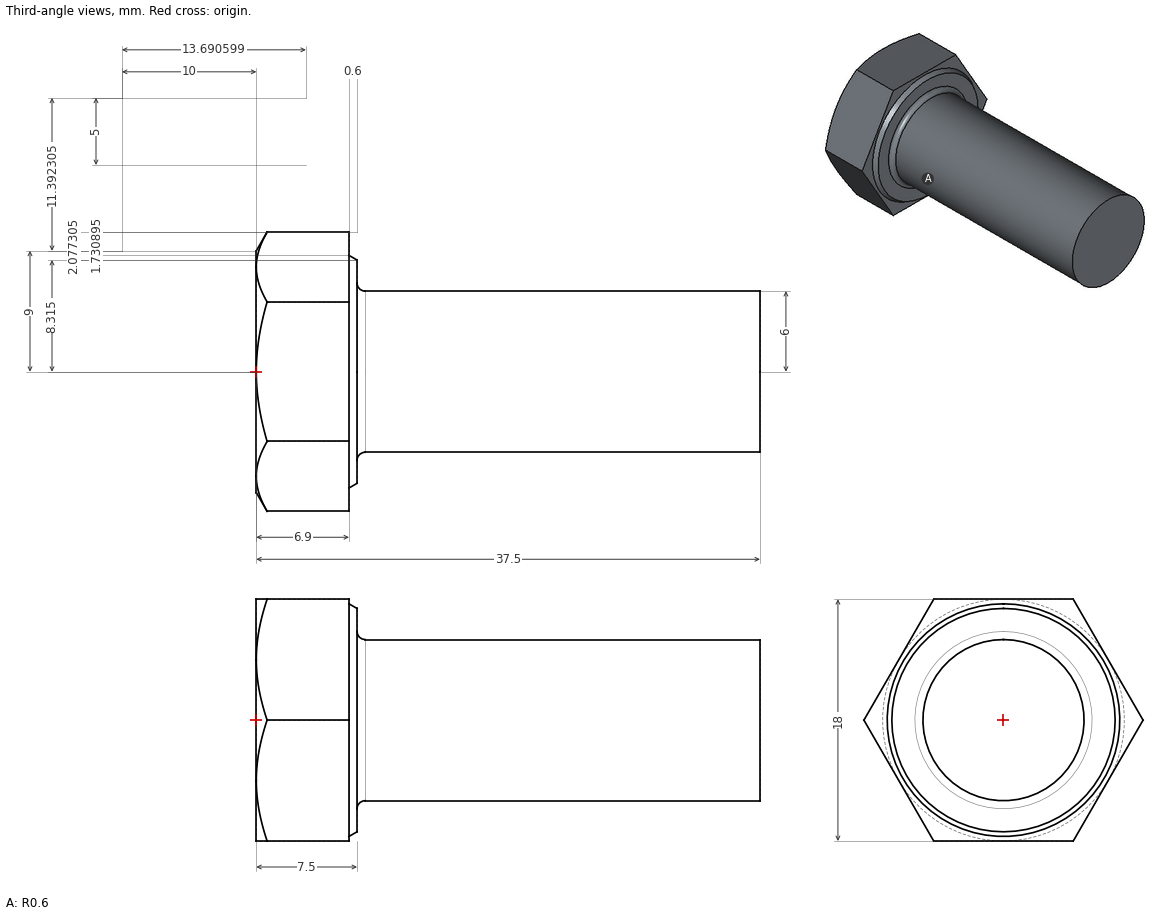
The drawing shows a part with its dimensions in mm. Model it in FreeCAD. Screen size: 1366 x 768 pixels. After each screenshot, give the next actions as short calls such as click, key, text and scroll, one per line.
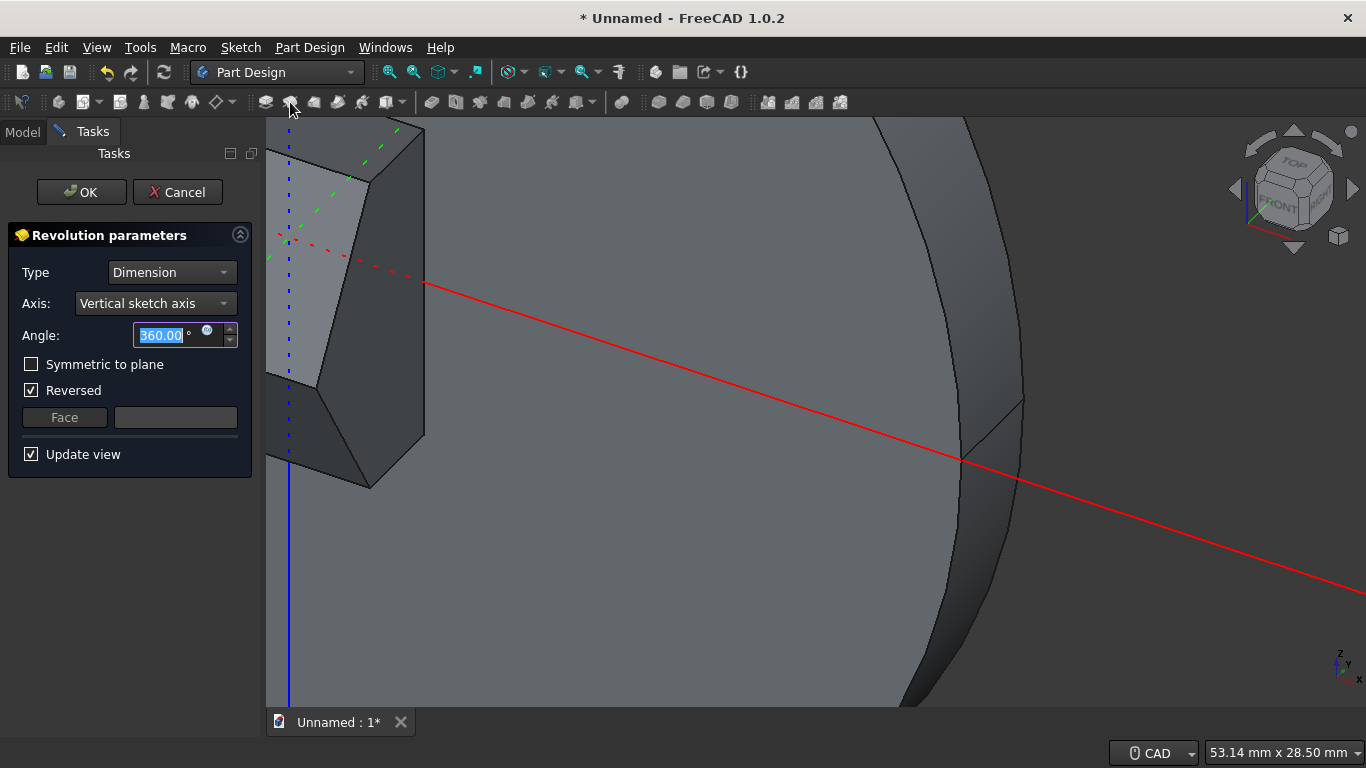
click(156, 304)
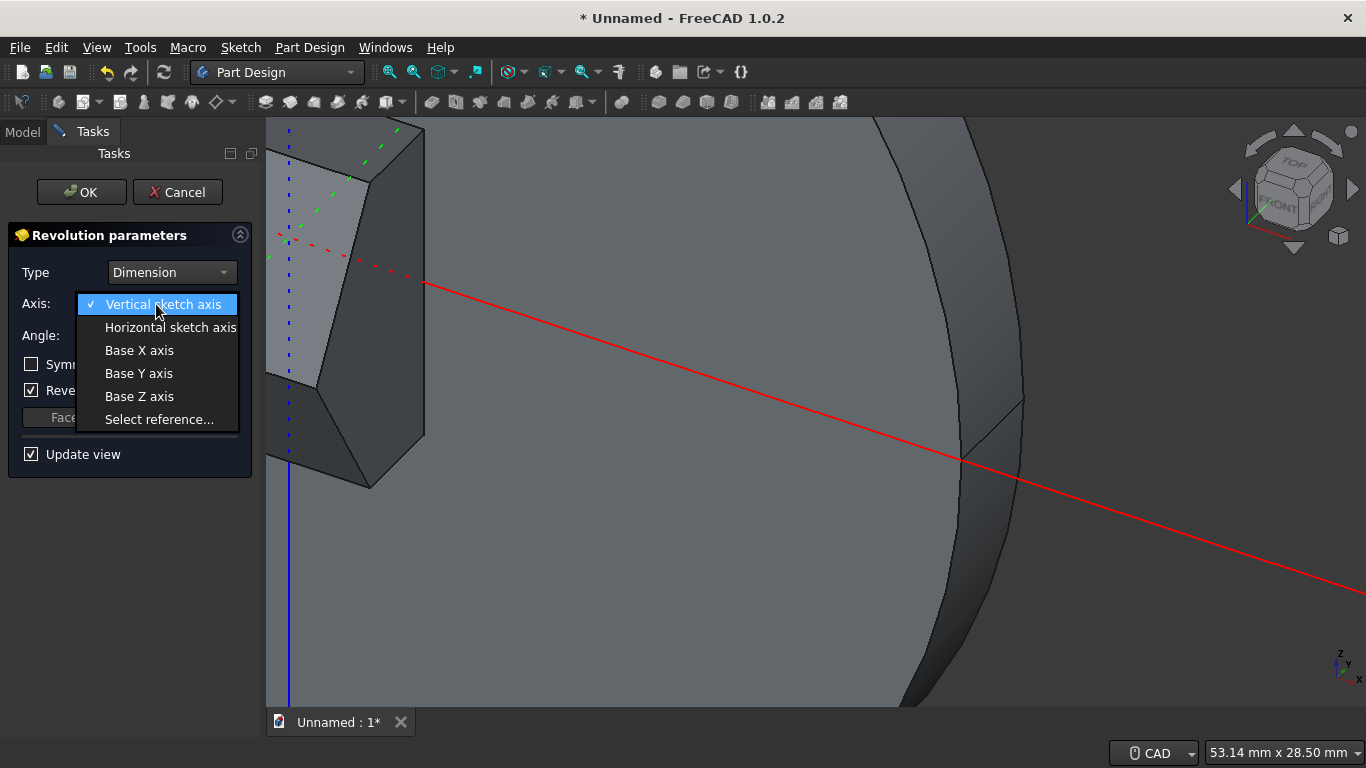
click(156, 328)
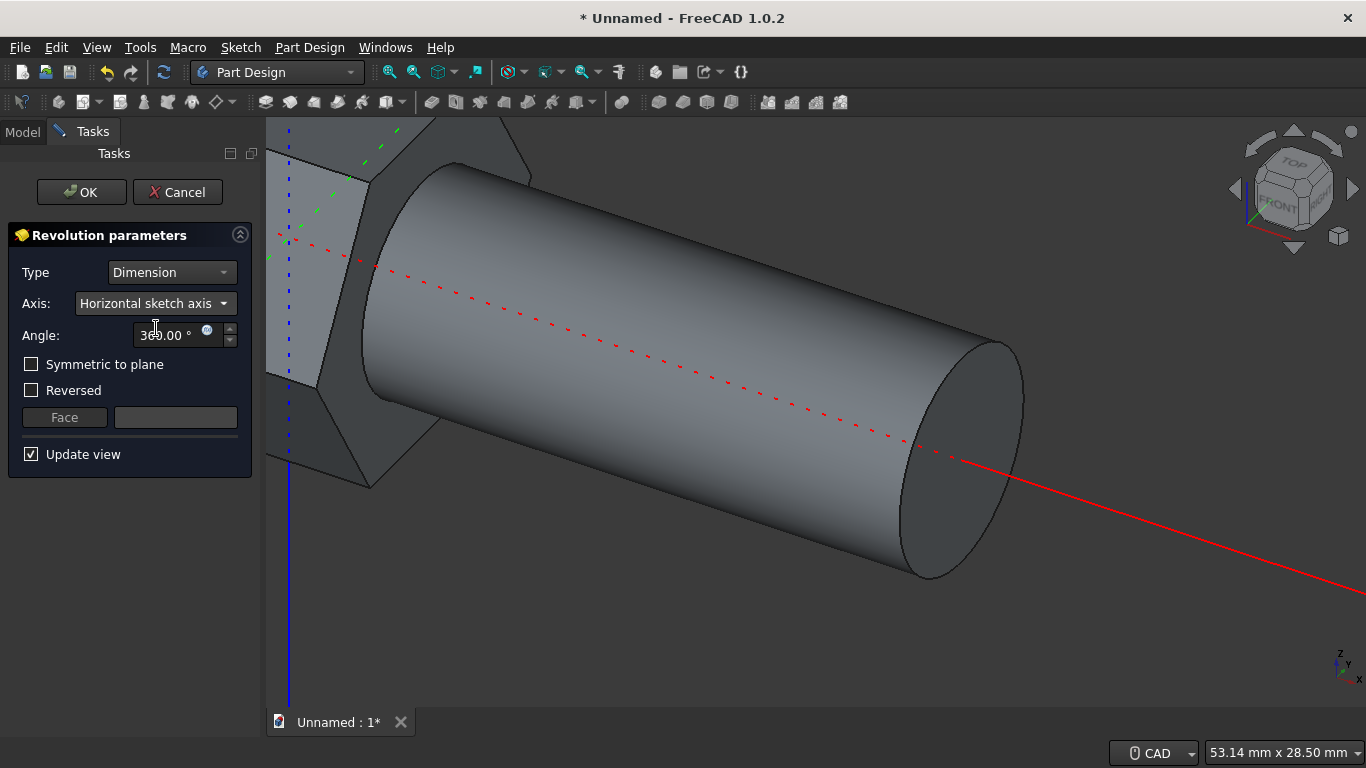
click(82, 192)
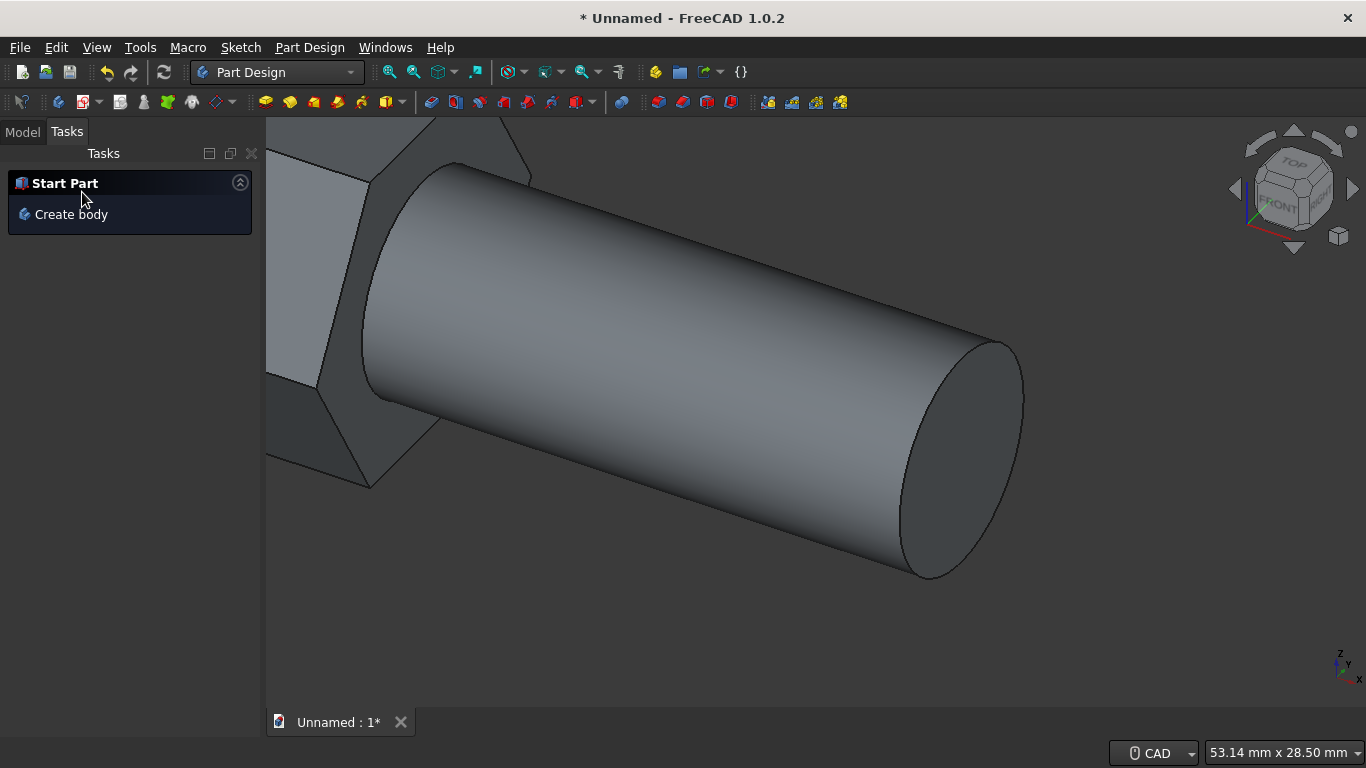
key(v)
key(f)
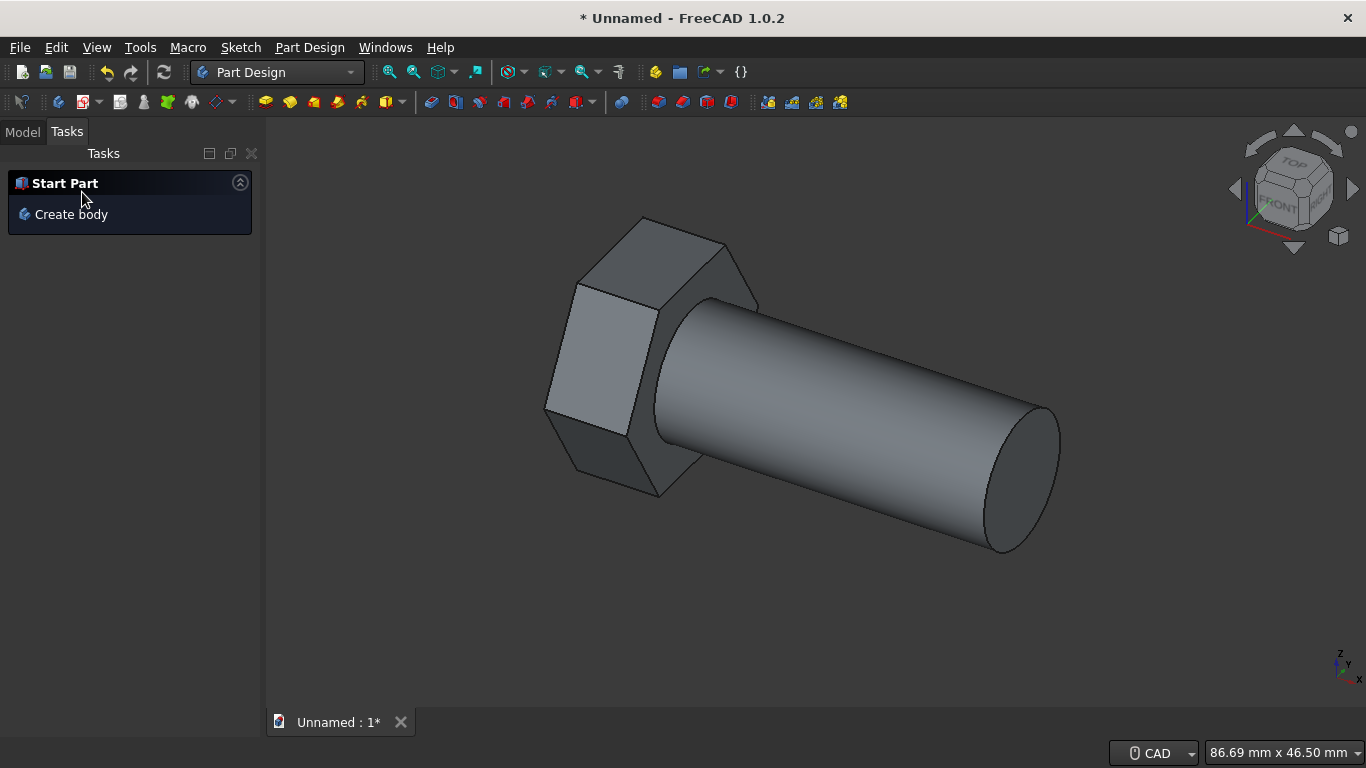
click(84, 102)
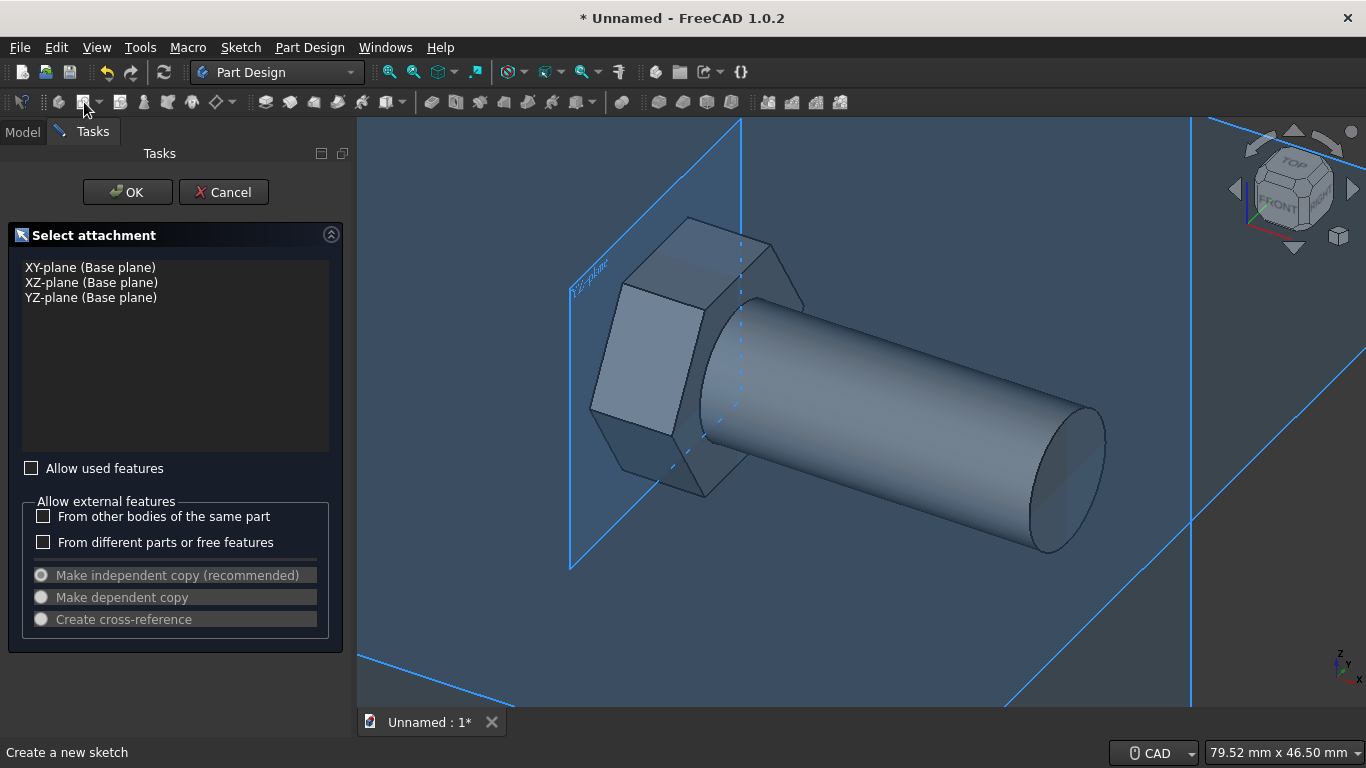
click(82, 268)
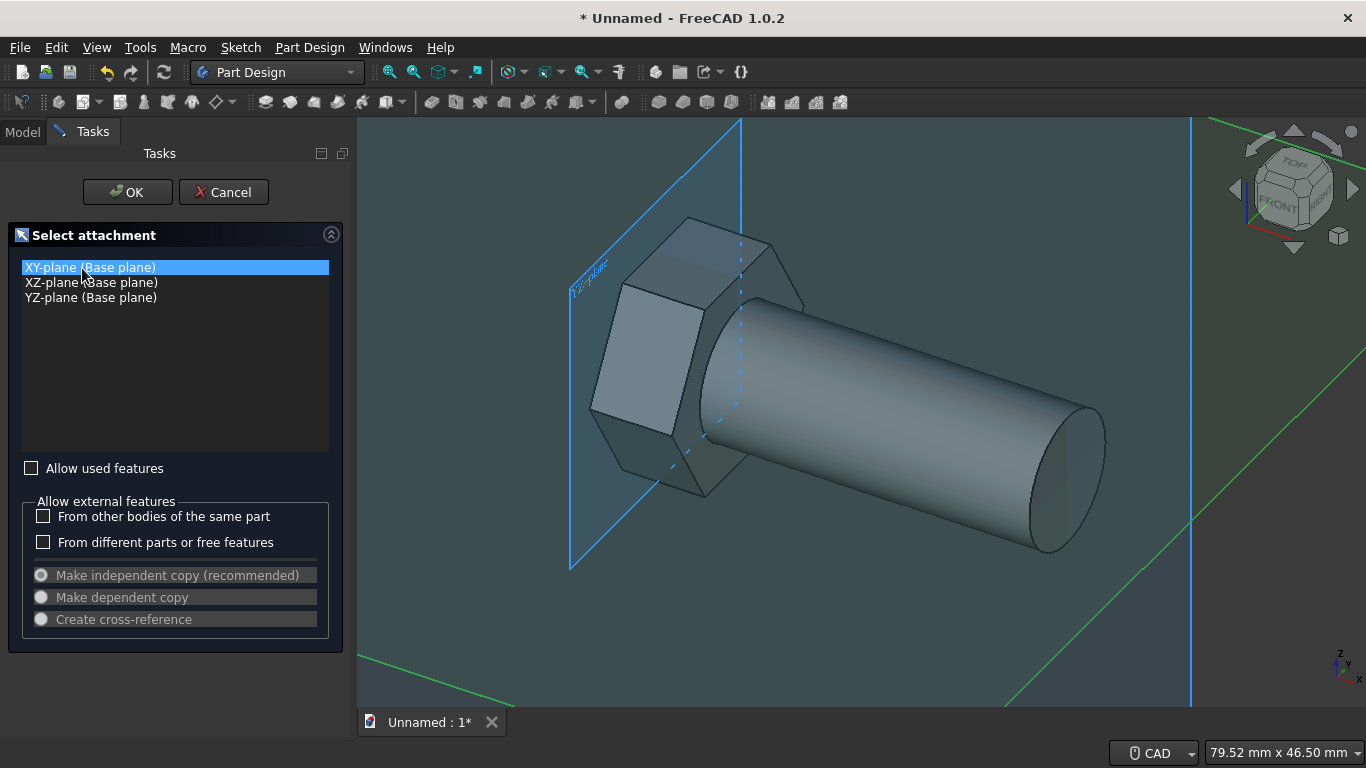
click(128, 192)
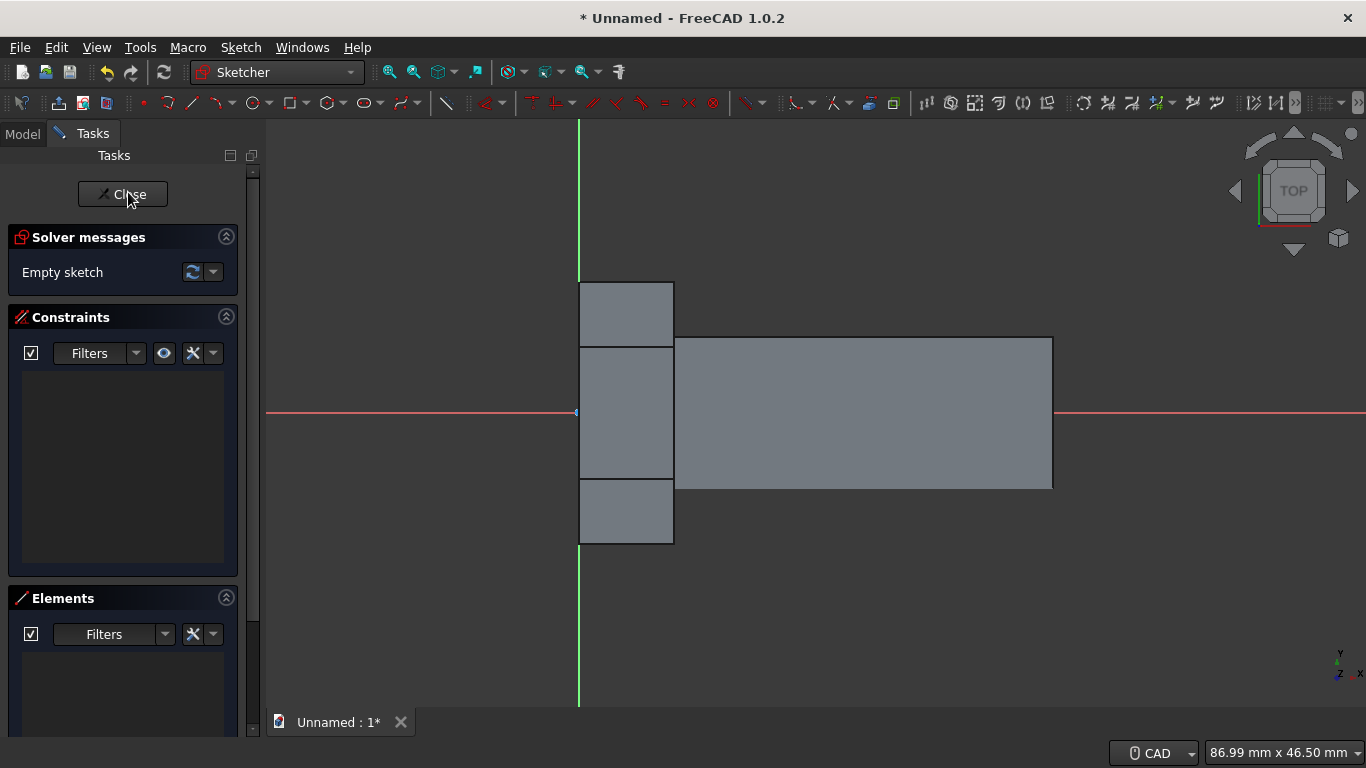
click(108, 104)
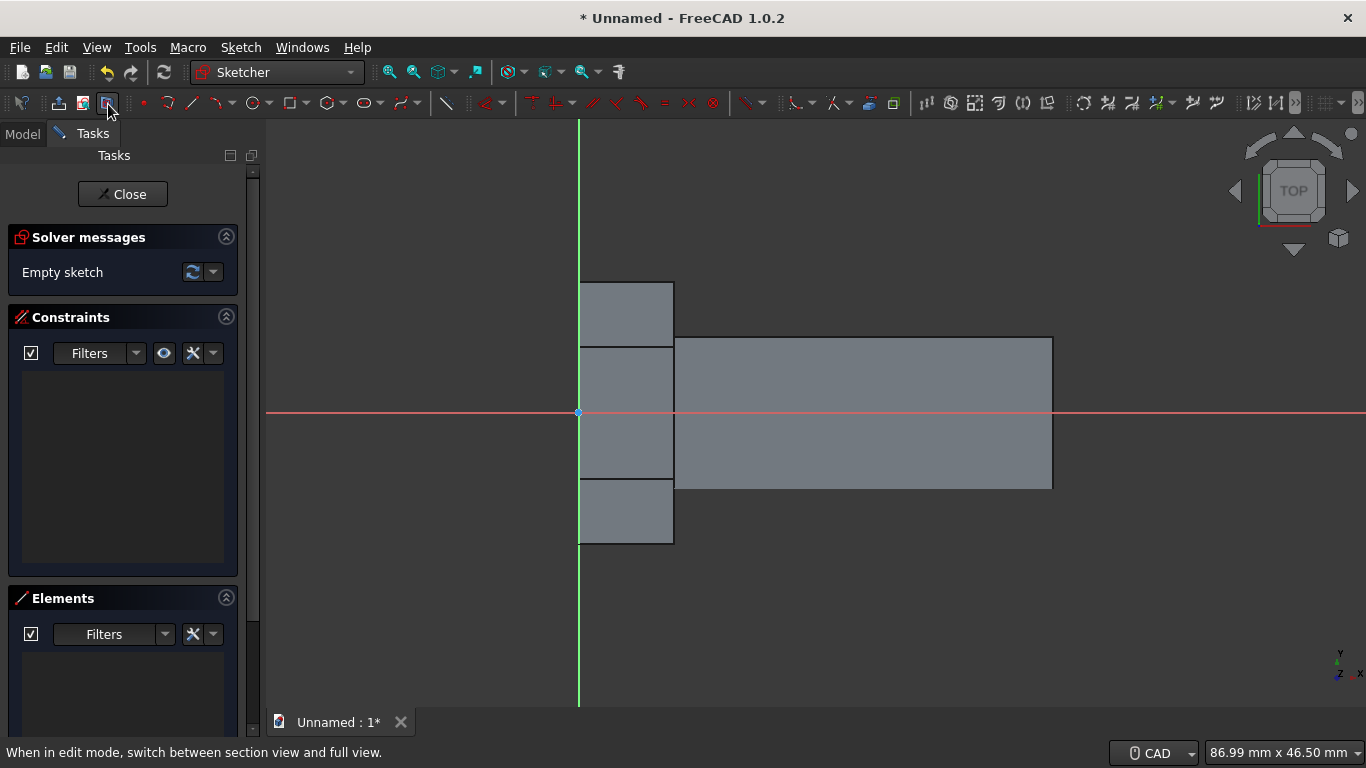
scroll(1201, 679, down, 1)